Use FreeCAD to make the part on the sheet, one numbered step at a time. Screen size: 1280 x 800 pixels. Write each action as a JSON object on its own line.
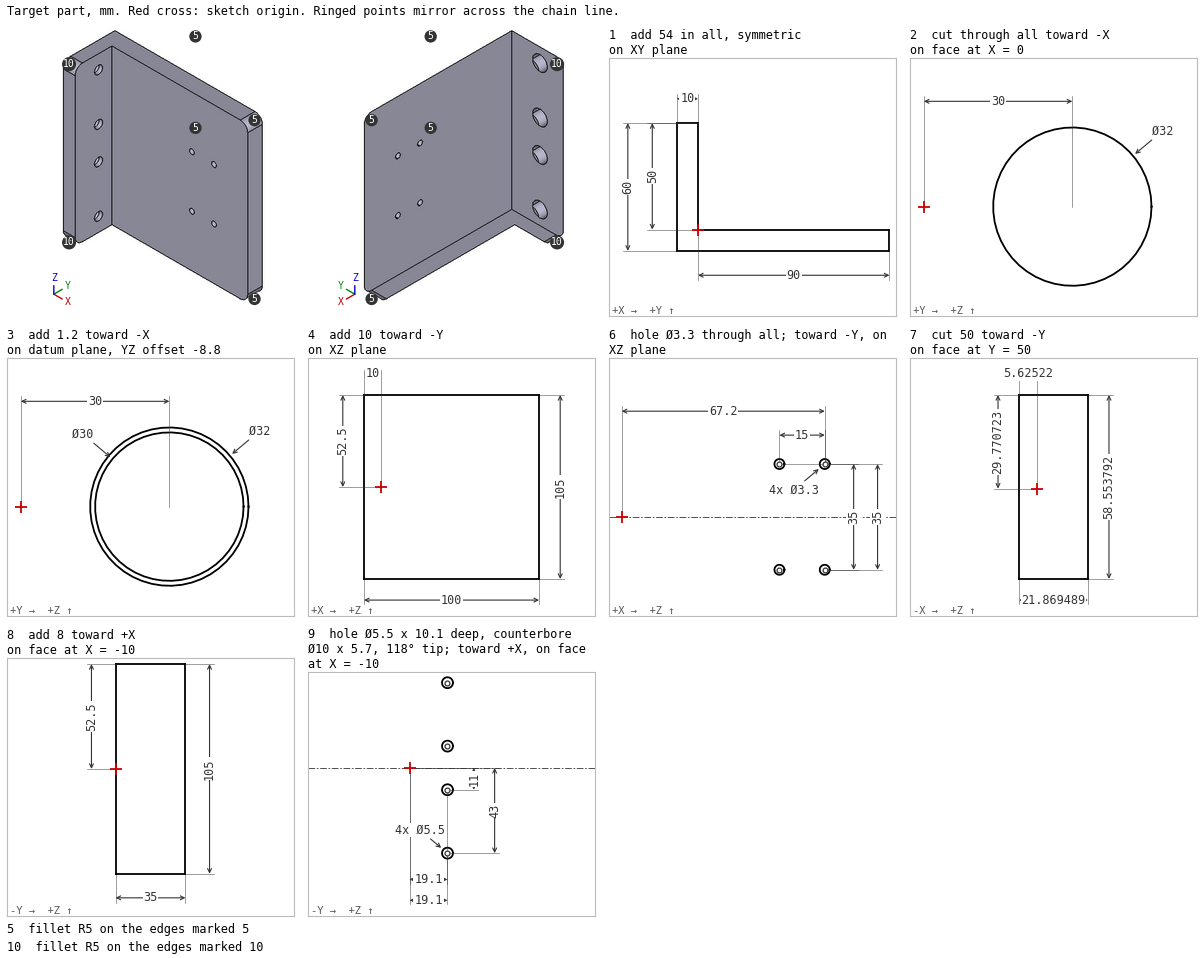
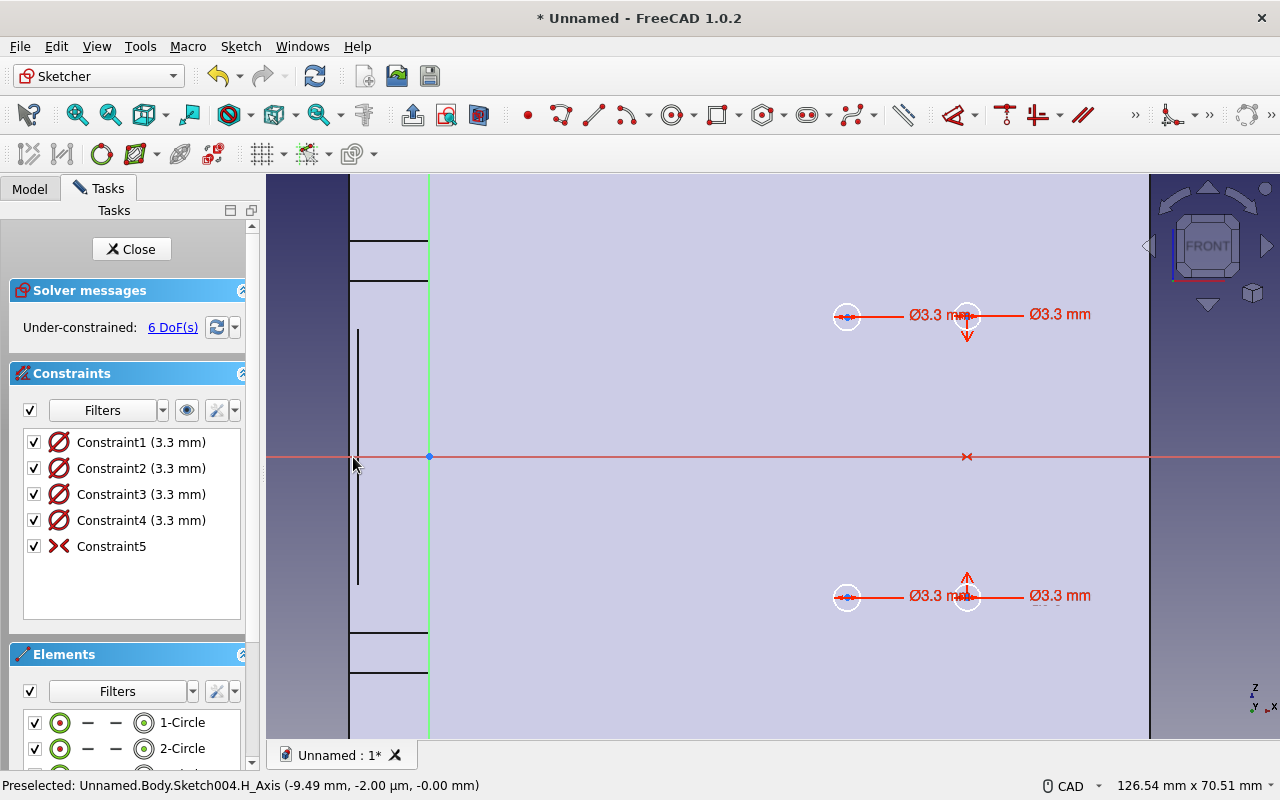
{"action": "left_click", "coordinate": [847, 317]}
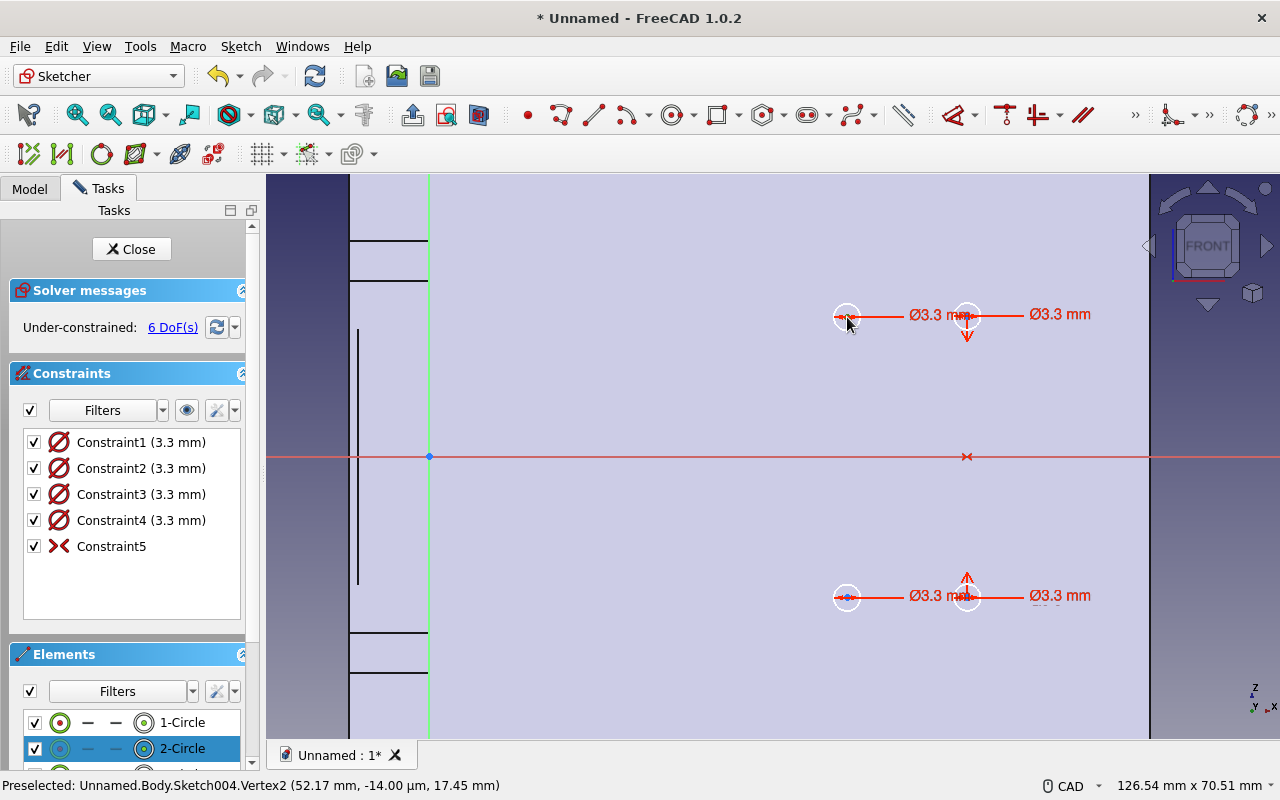
{"action": "left_click", "coordinate": [847, 598]}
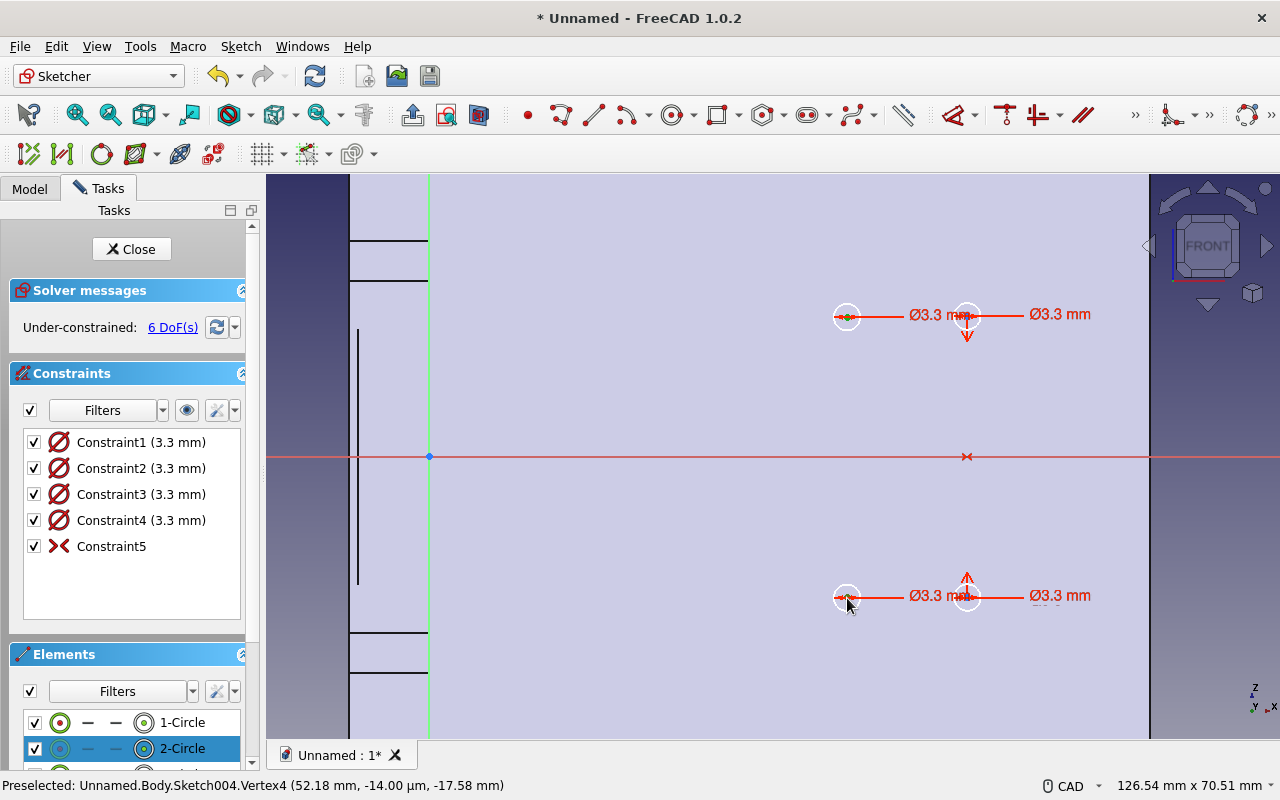
{"action": "left_click", "coordinate": [353, 457]}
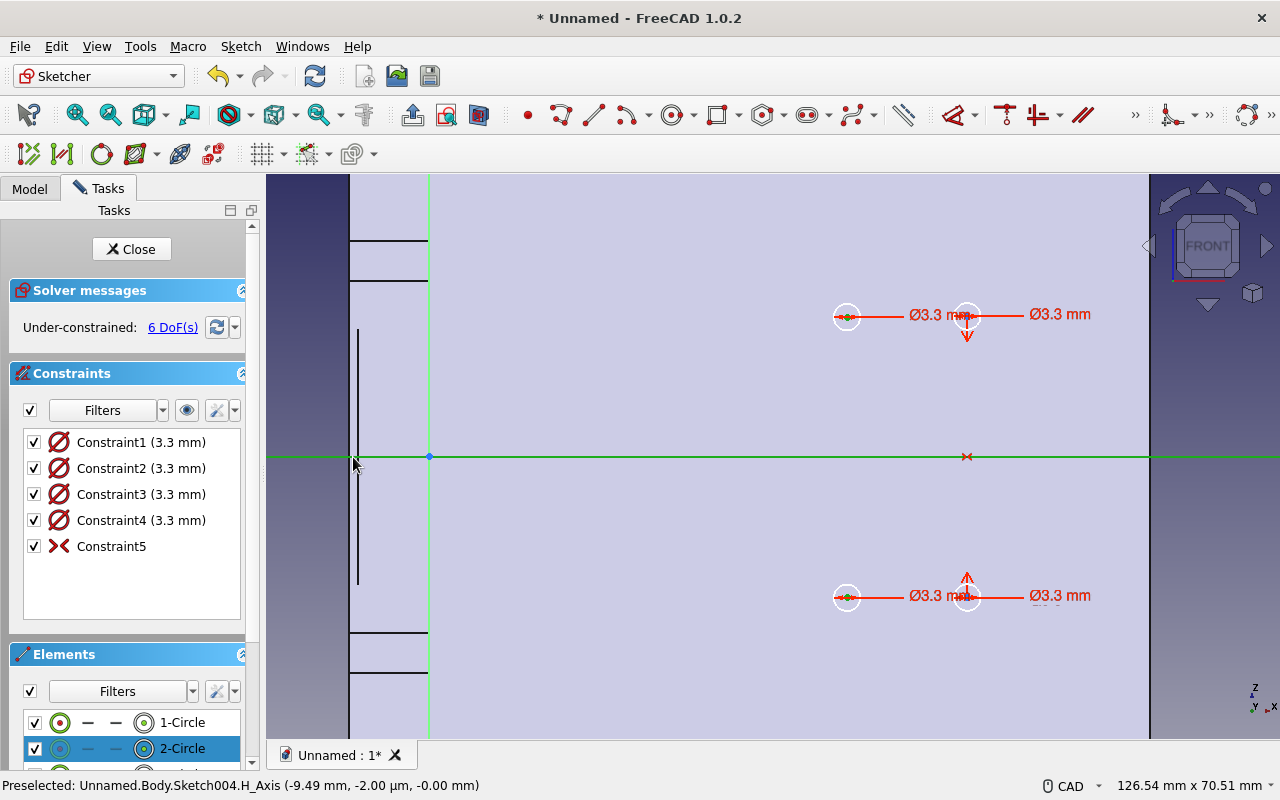
{"action": "key", "text": "s"}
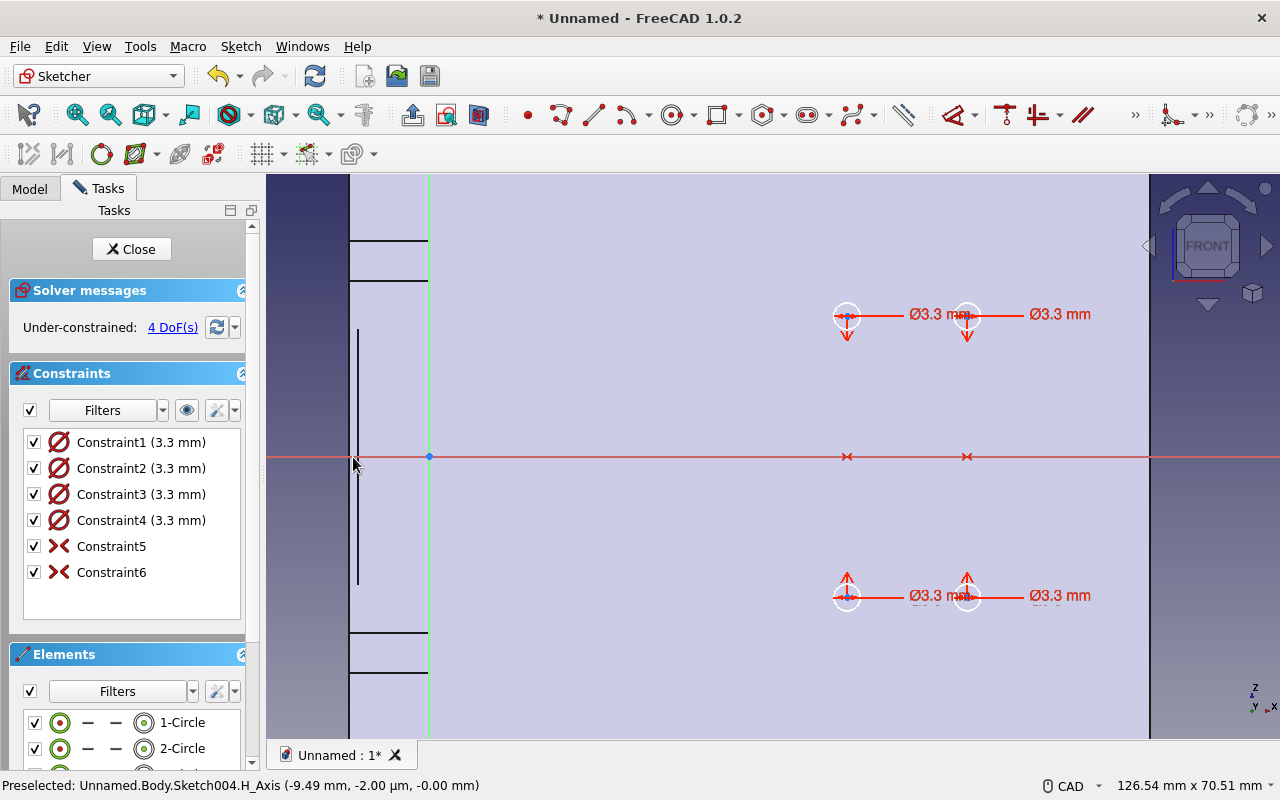
{"action": "left_click", "coordinate": [952, 116]}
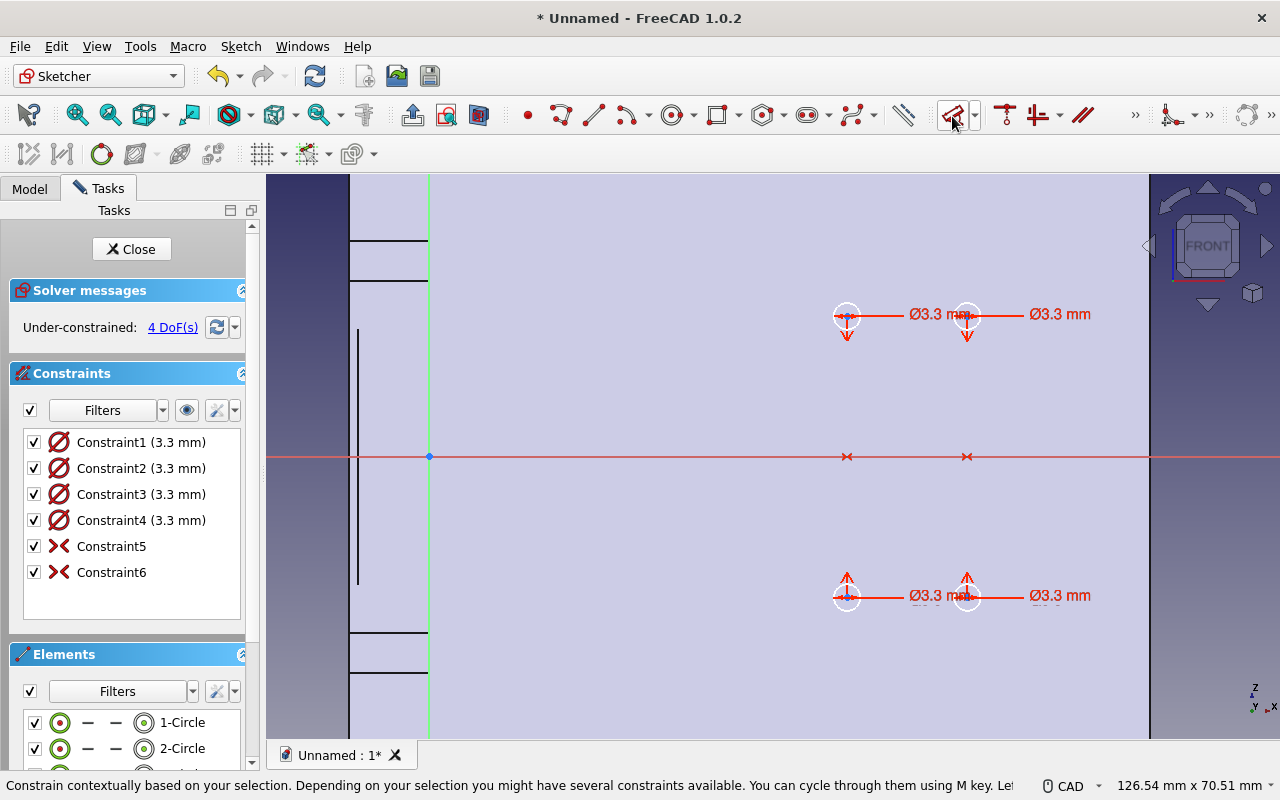
{"action": "left_click", "coordinate": [967, 316]}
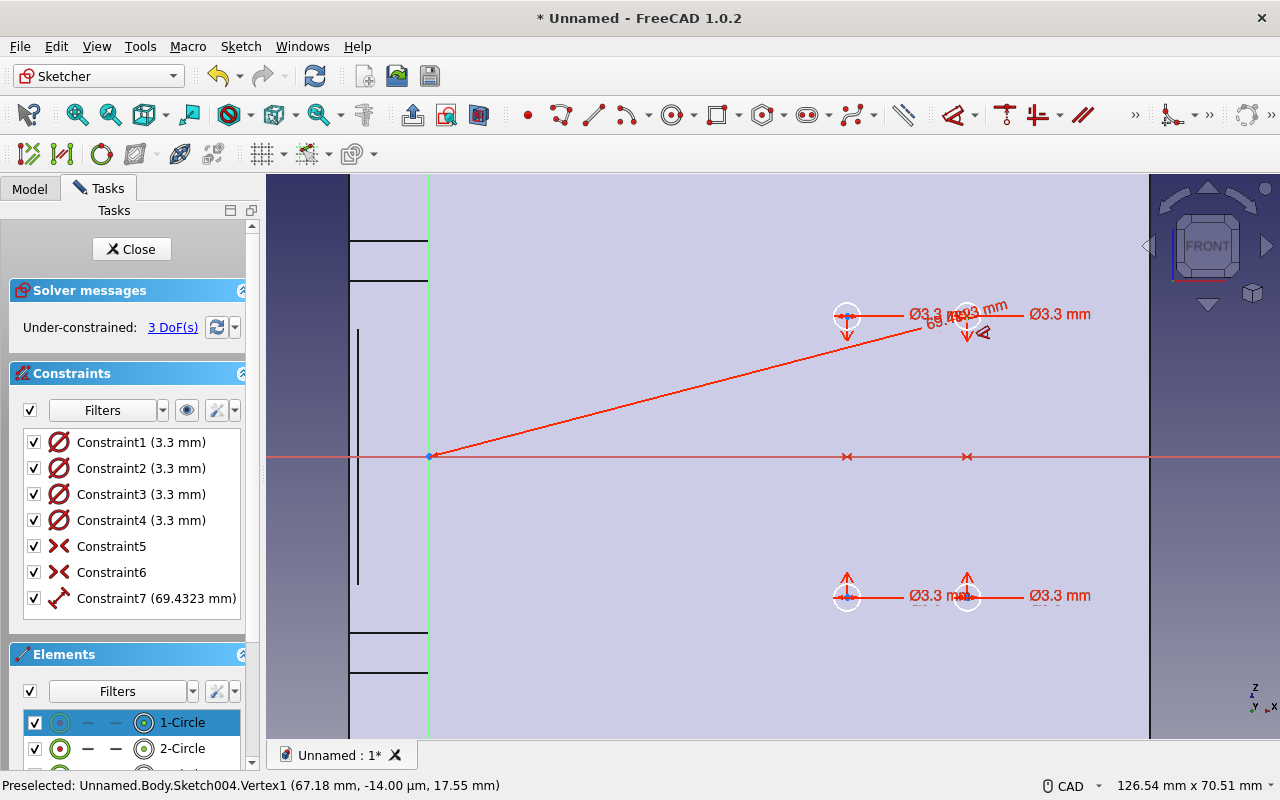
{"action": "left_click", "coordinate": [847, 316]}
{"action": "left_click", "coordinate": [907, 282]}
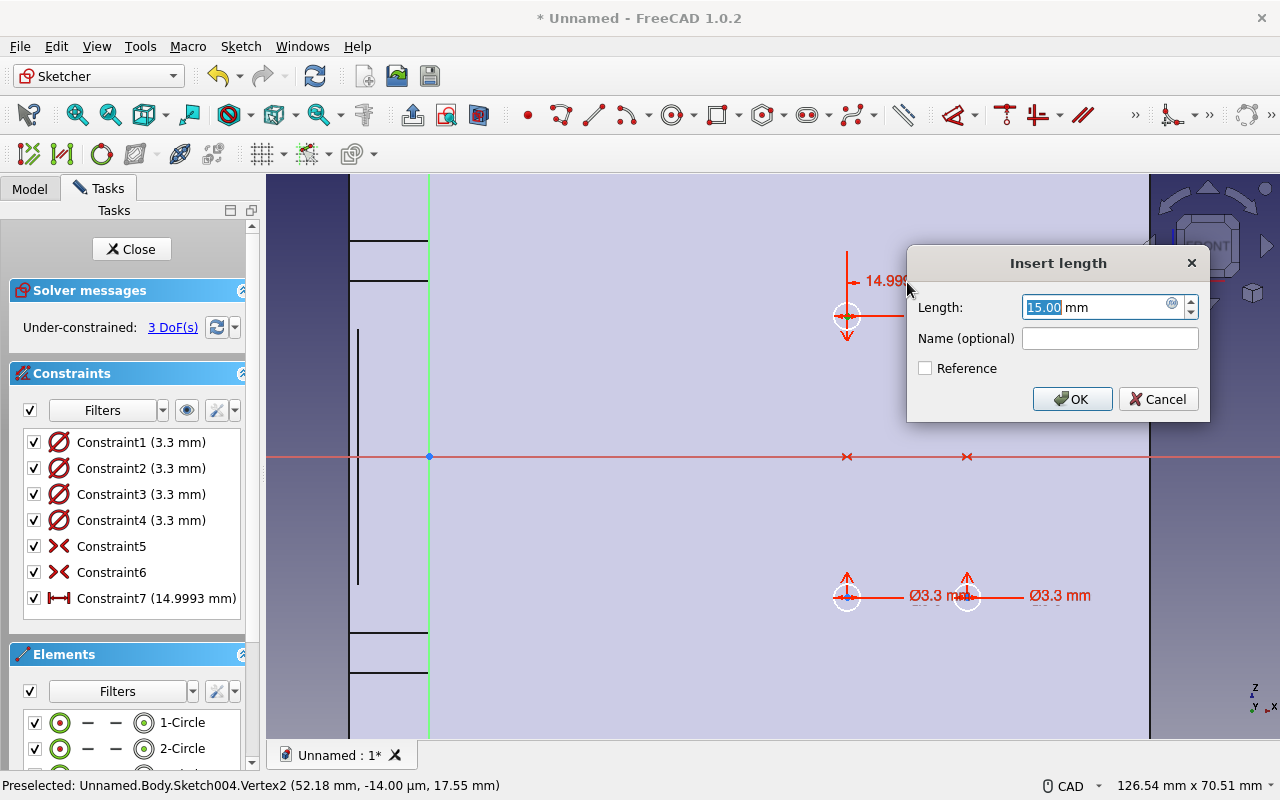
{"action": "type", "text": "15"}
{"action": "key", "text": "Return"}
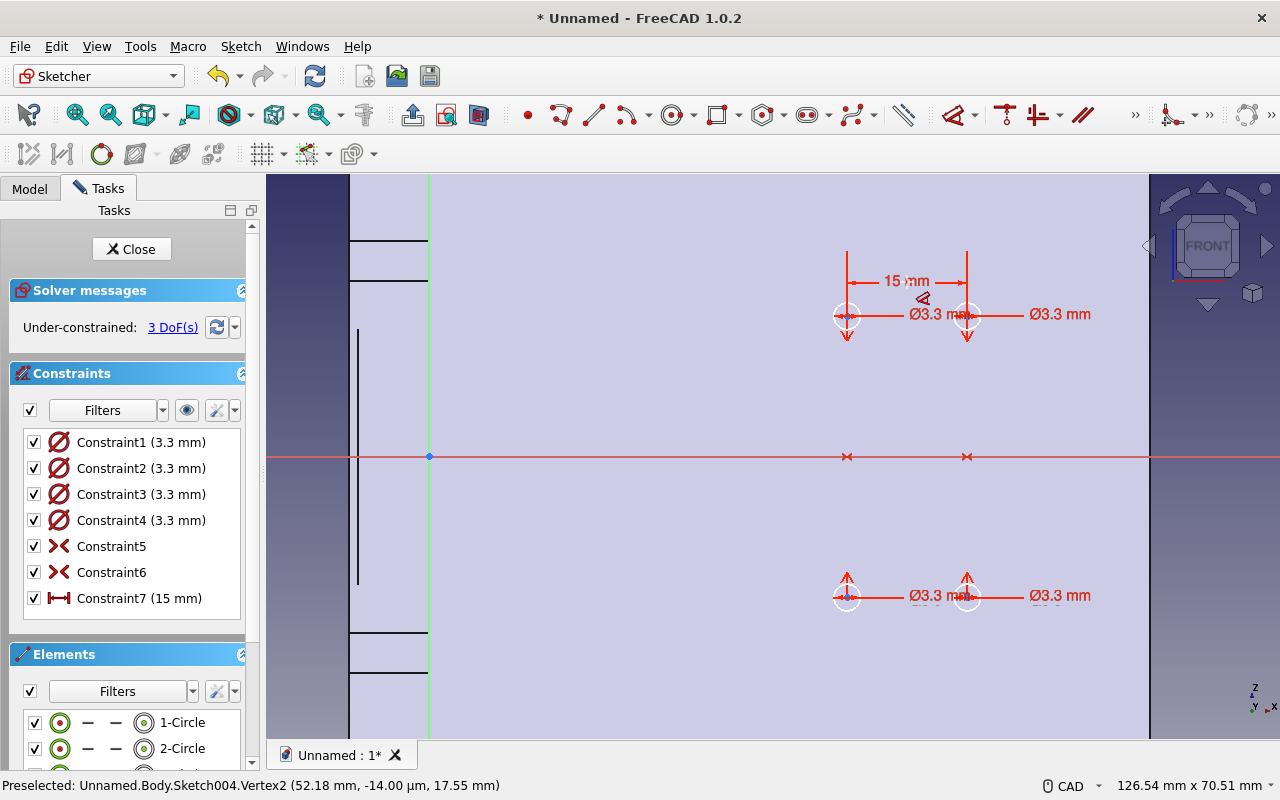
{"action": "left_click", "coordinate": [967, 316]}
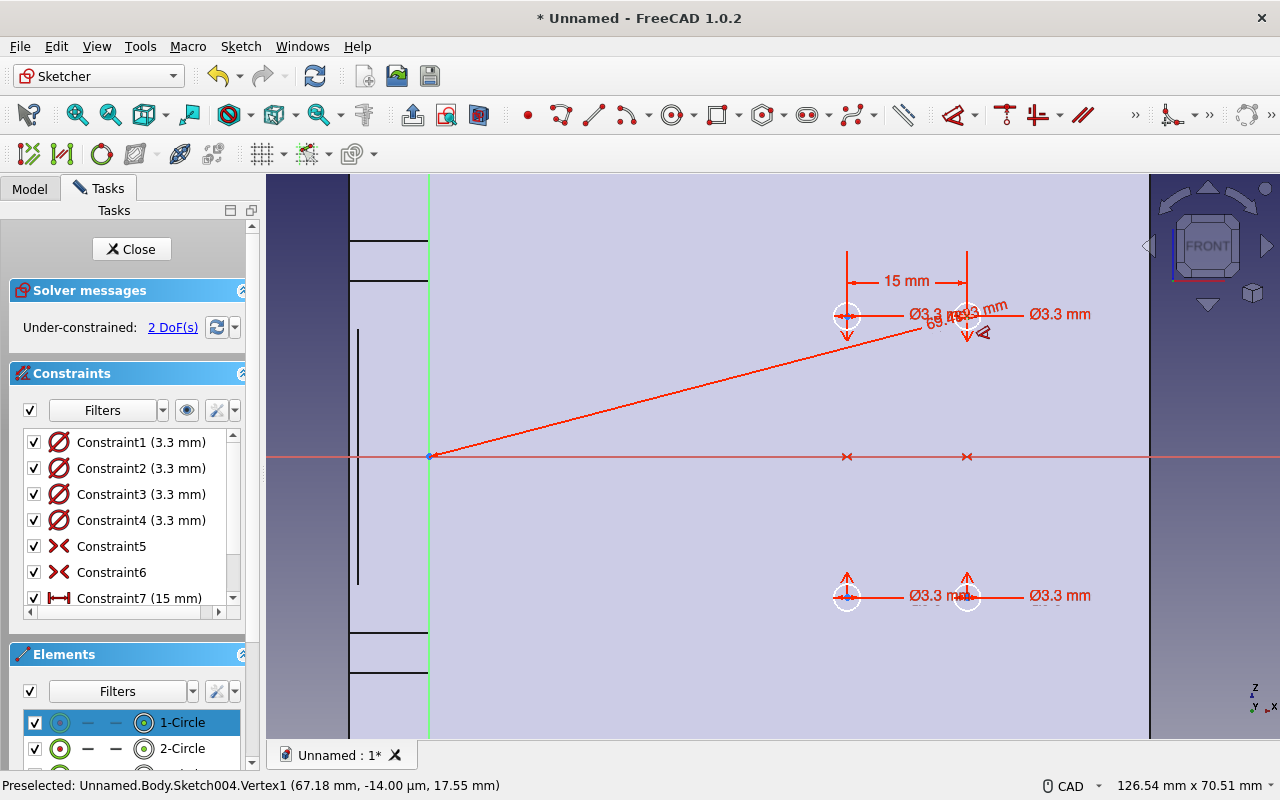
{"action": "left_click", "coordinate": [967, 598]}
{"action": "left_click", "coordinate": [1001, 392]}